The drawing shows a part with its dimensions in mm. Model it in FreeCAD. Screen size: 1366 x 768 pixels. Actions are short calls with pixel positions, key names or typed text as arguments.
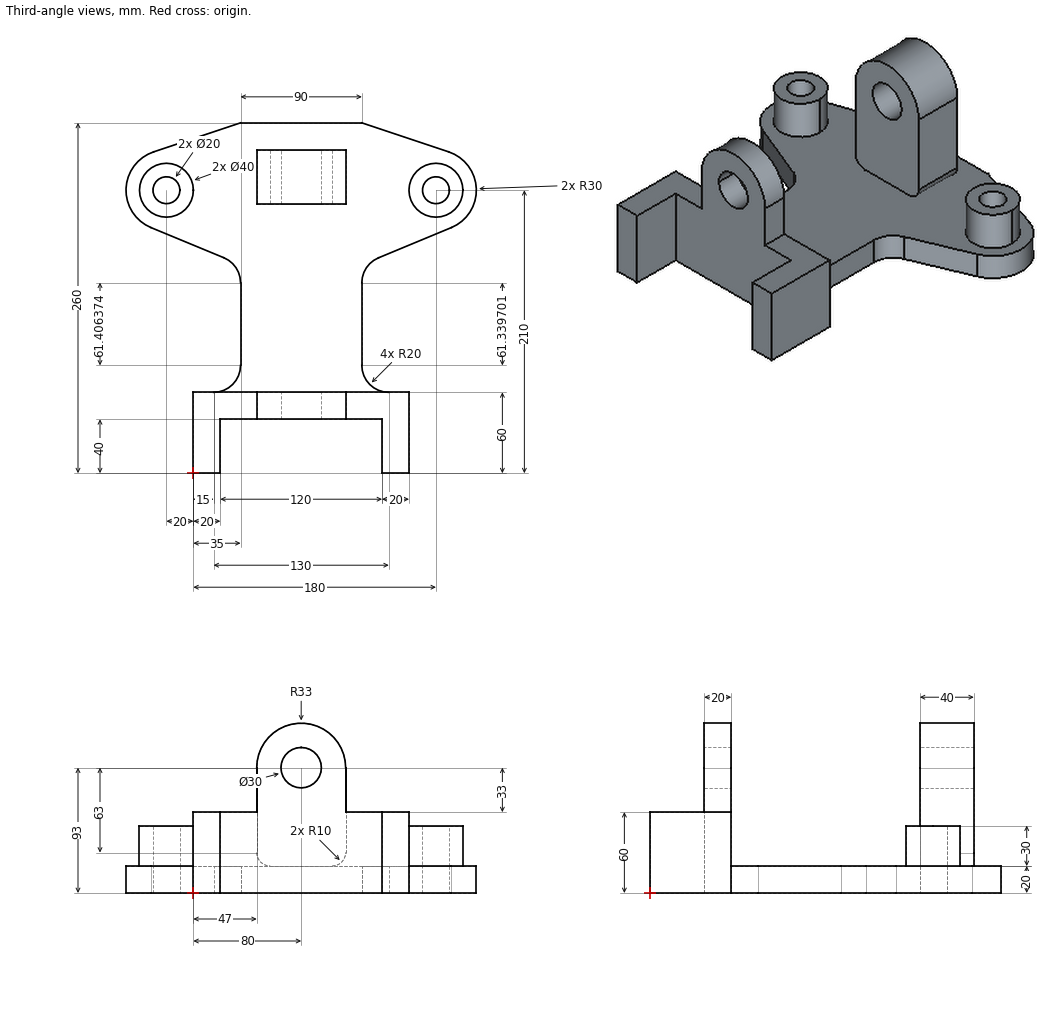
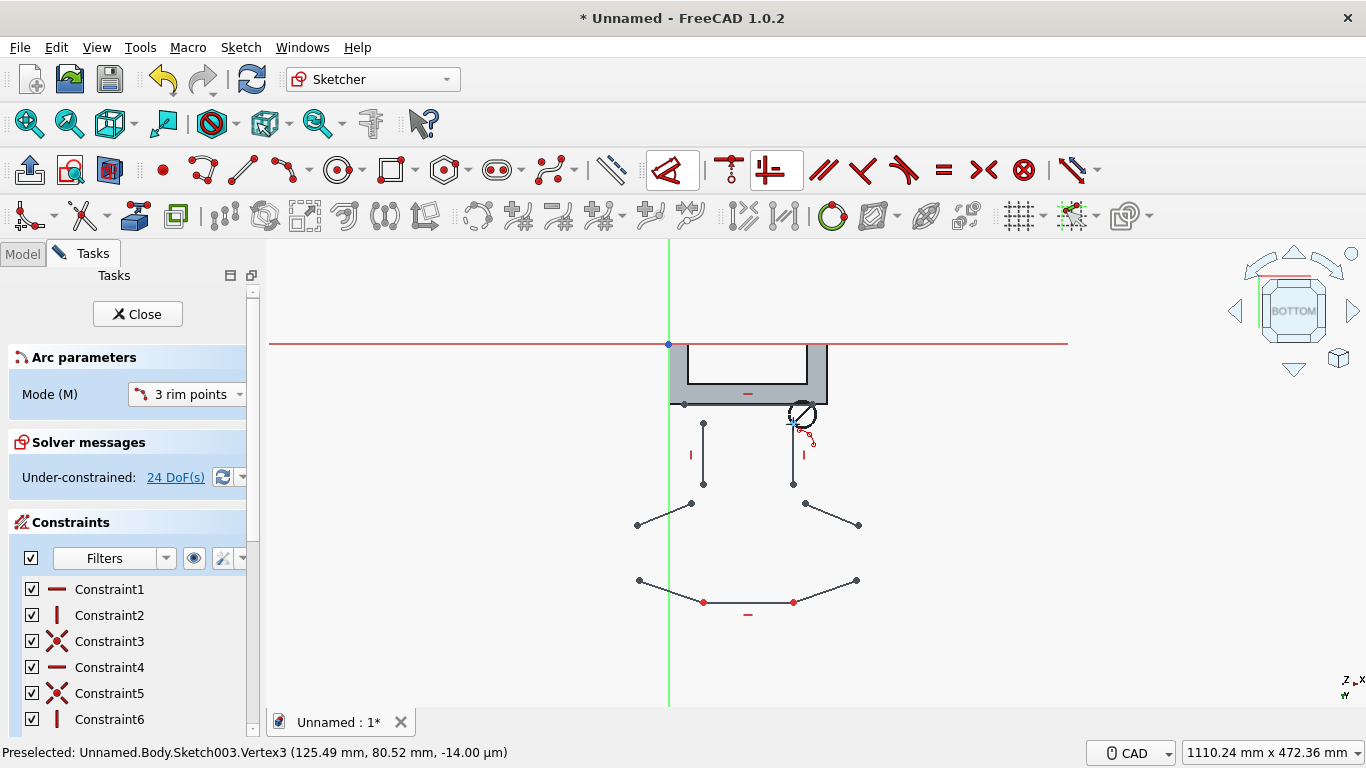
scroll(798, 409, up, 6)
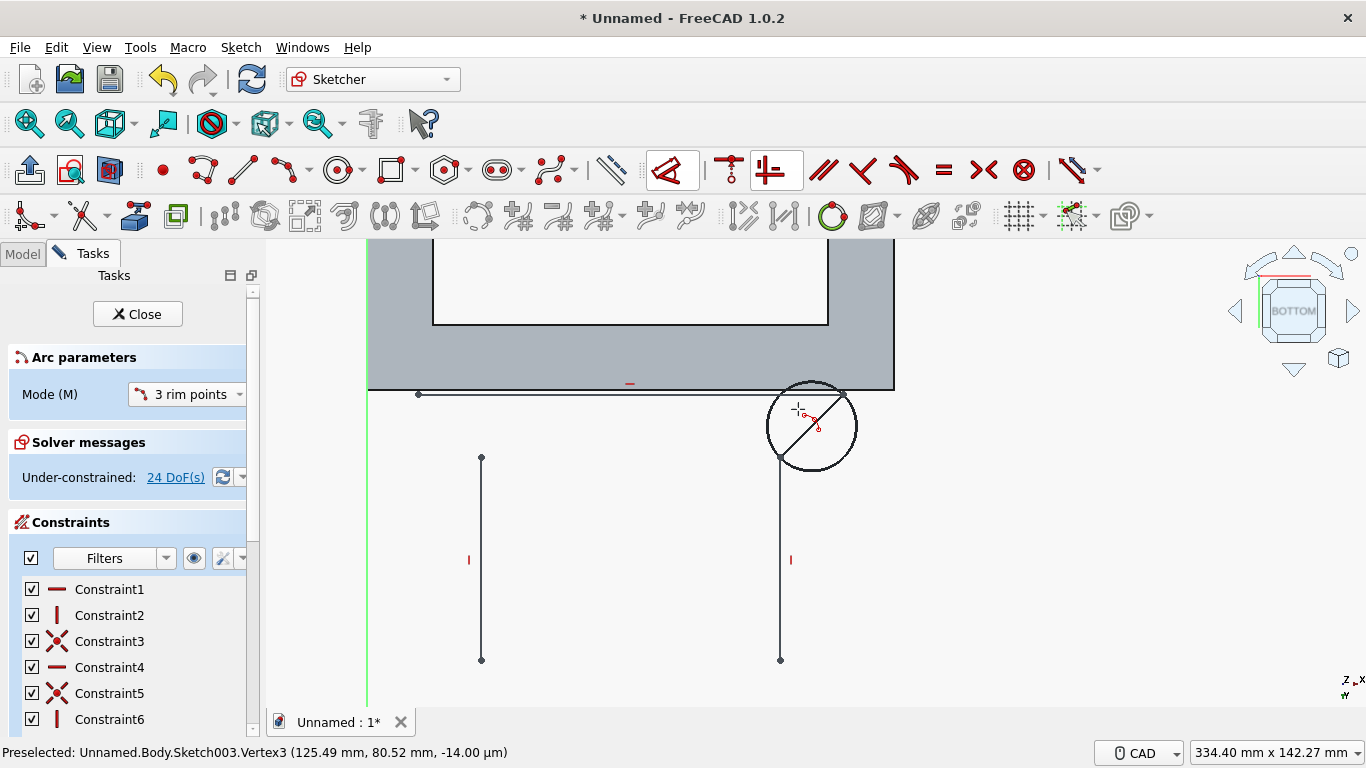
click(798, 410)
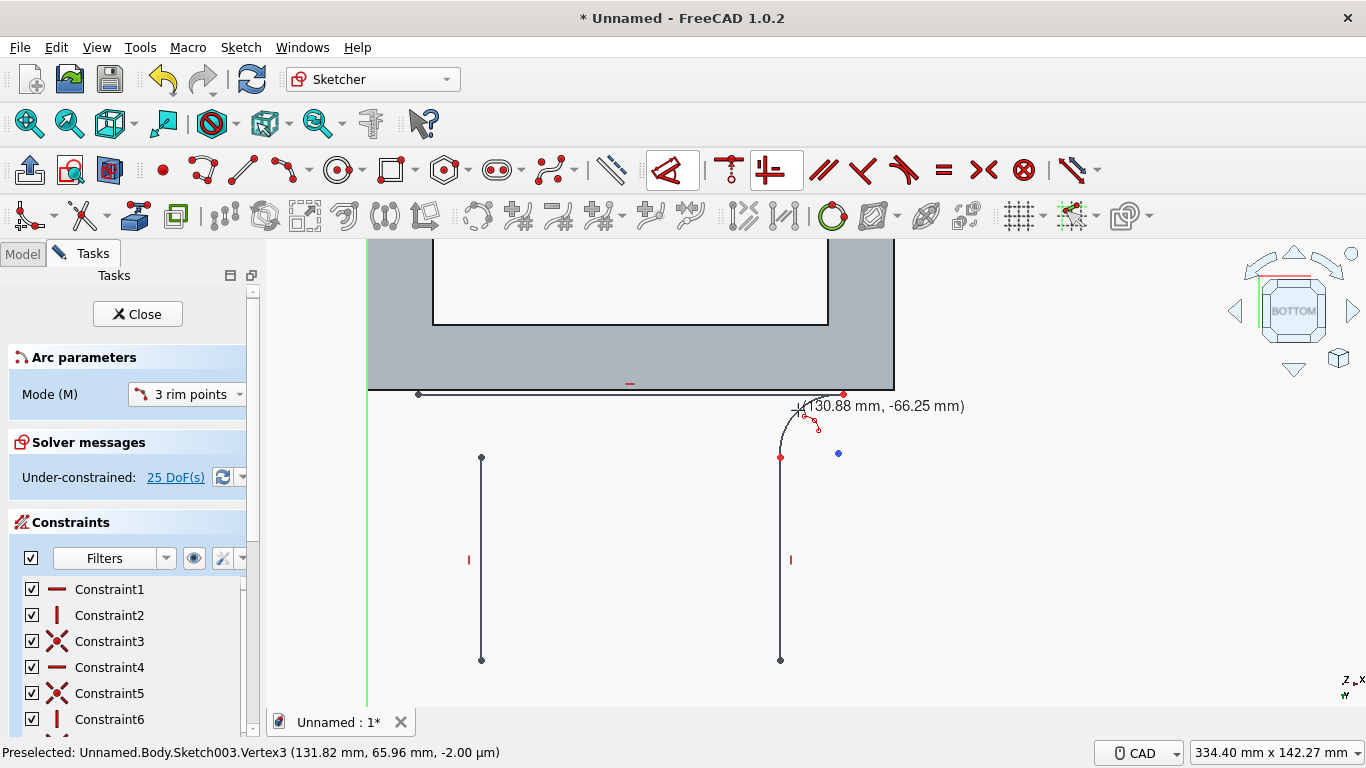
click(780, 660)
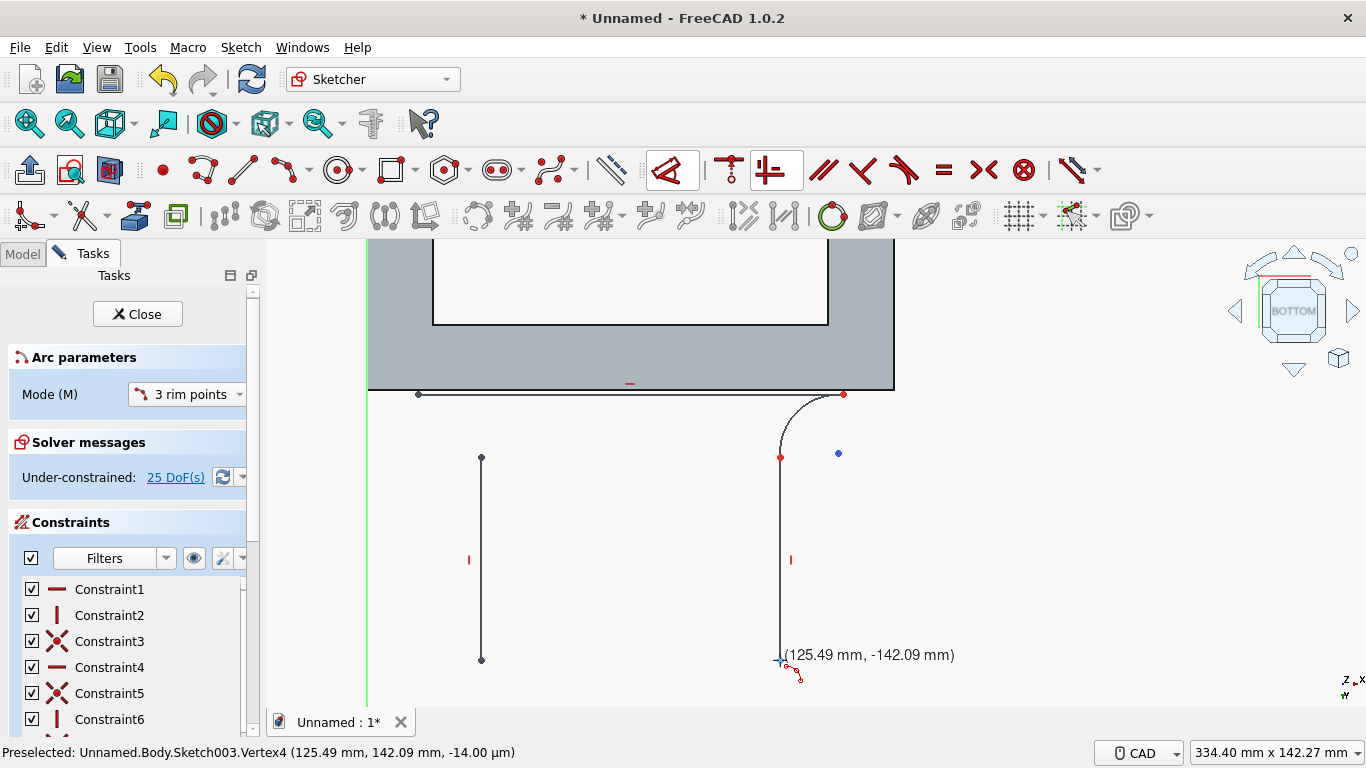
scroll(816, 387, down, 5)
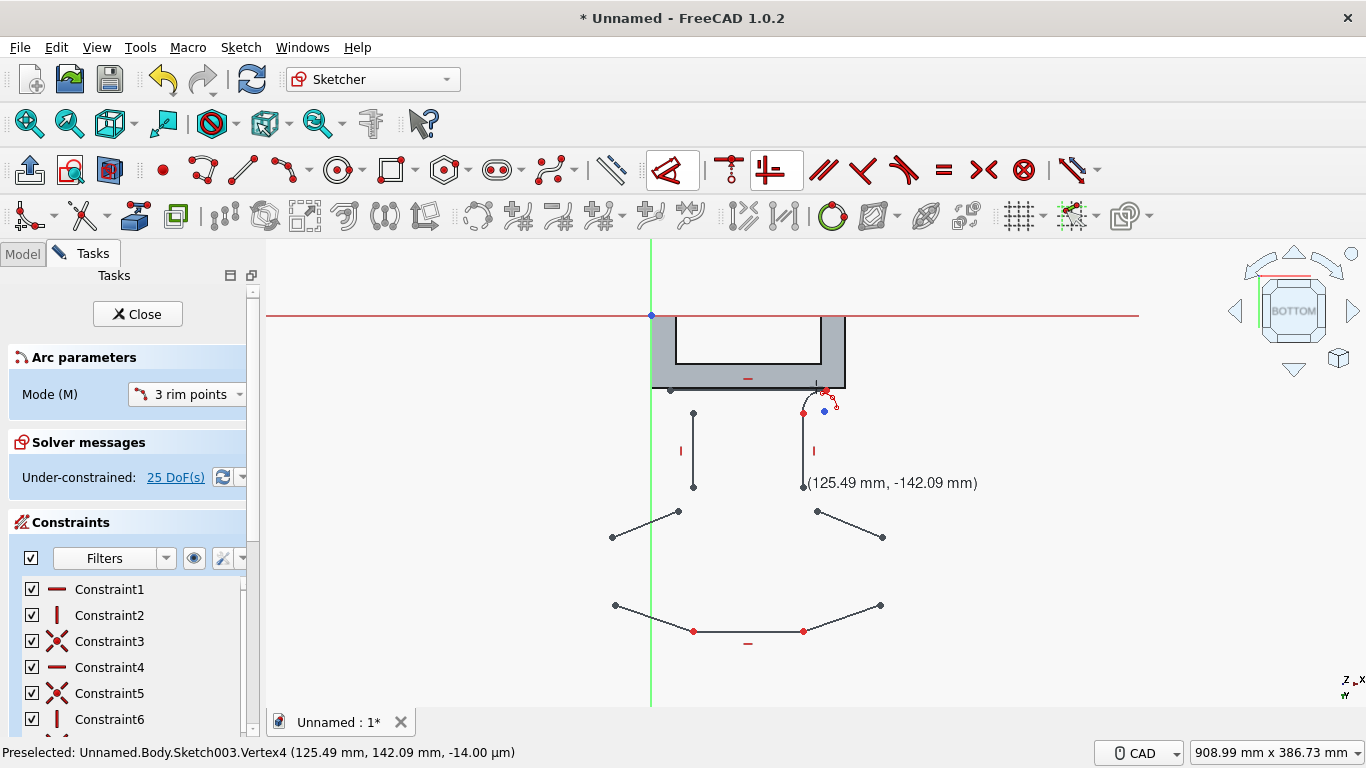
click(818, 511)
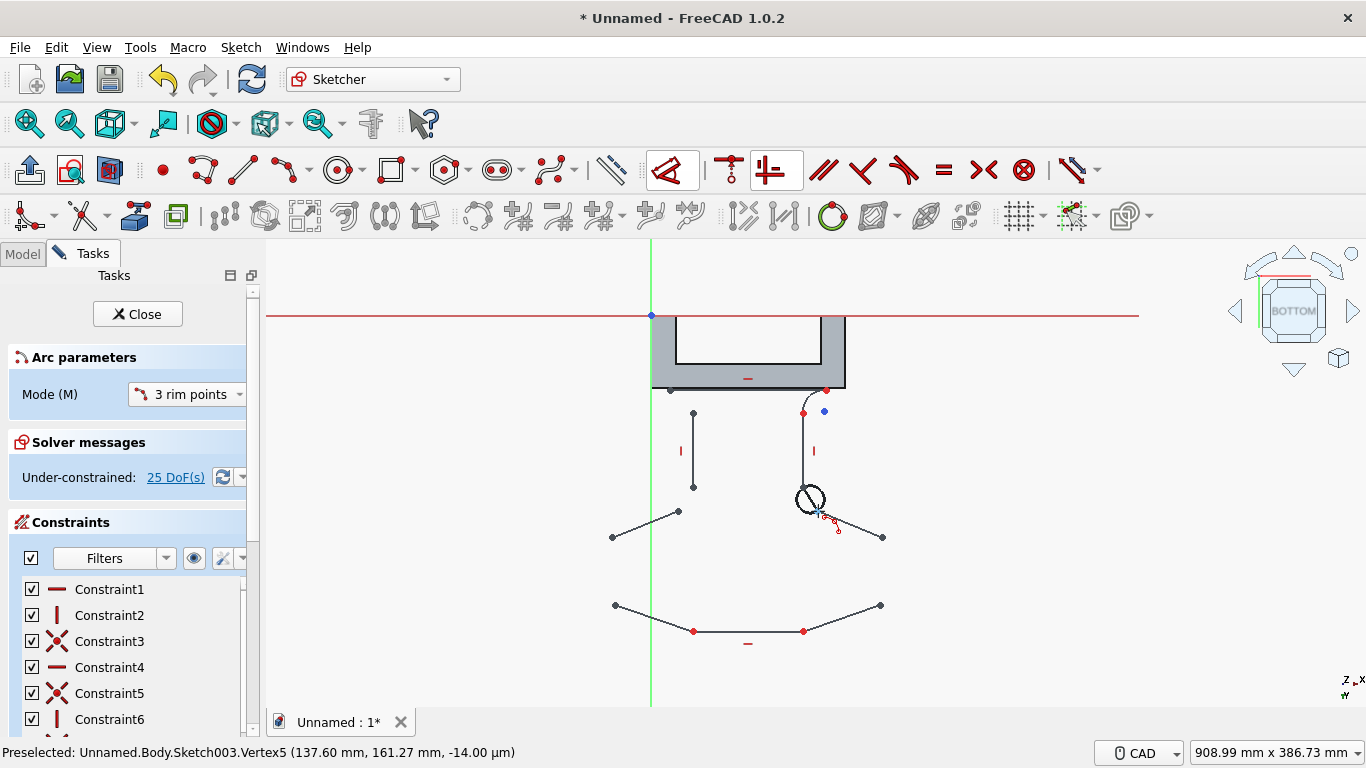
scroll(807, 500, up, 7)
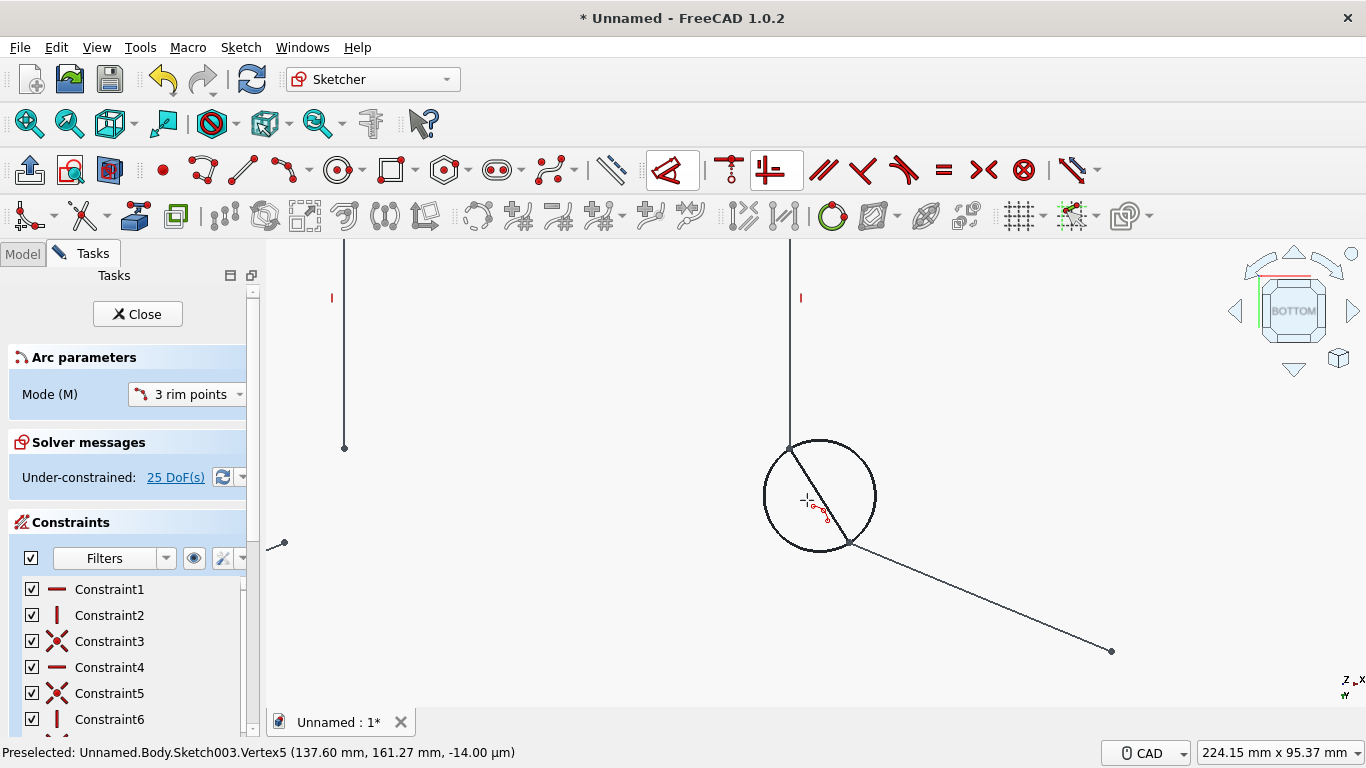
click(804, 500)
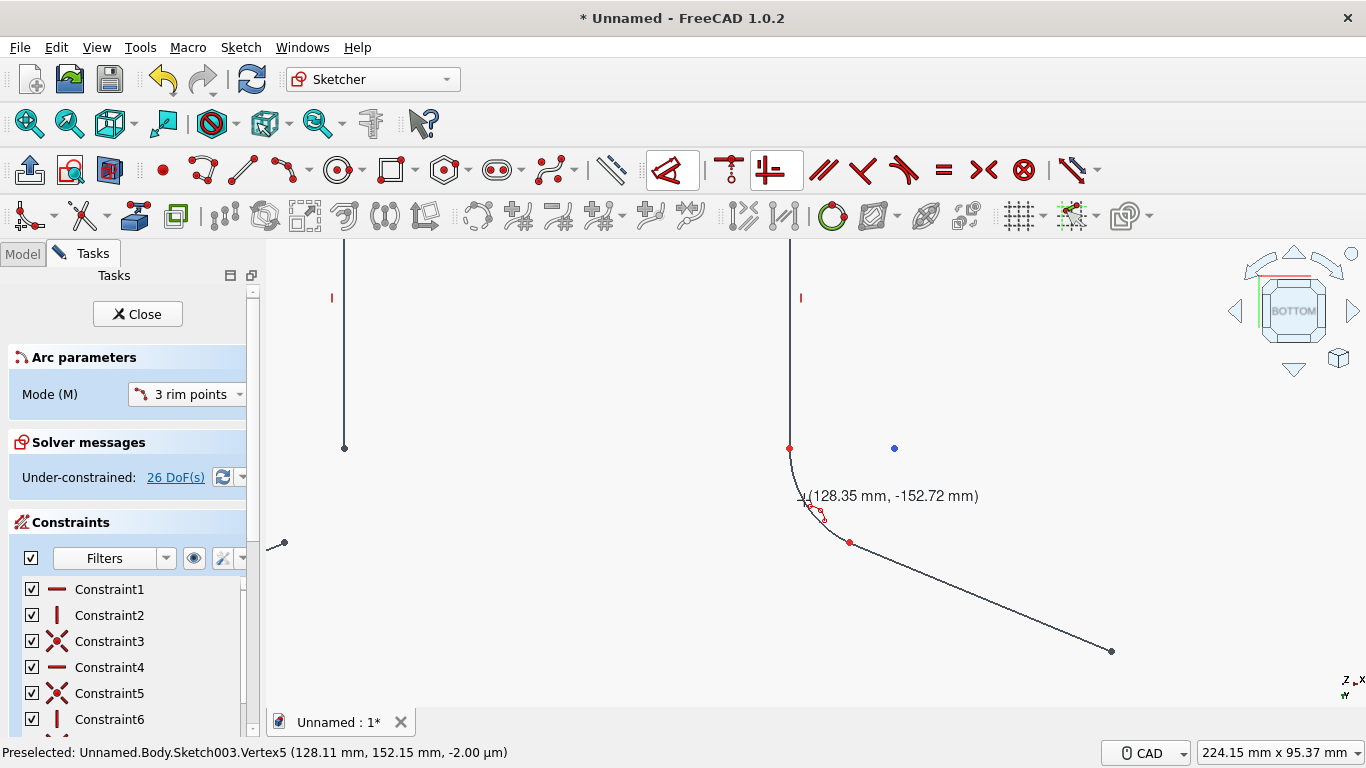
scroll(807, 500, down, 7)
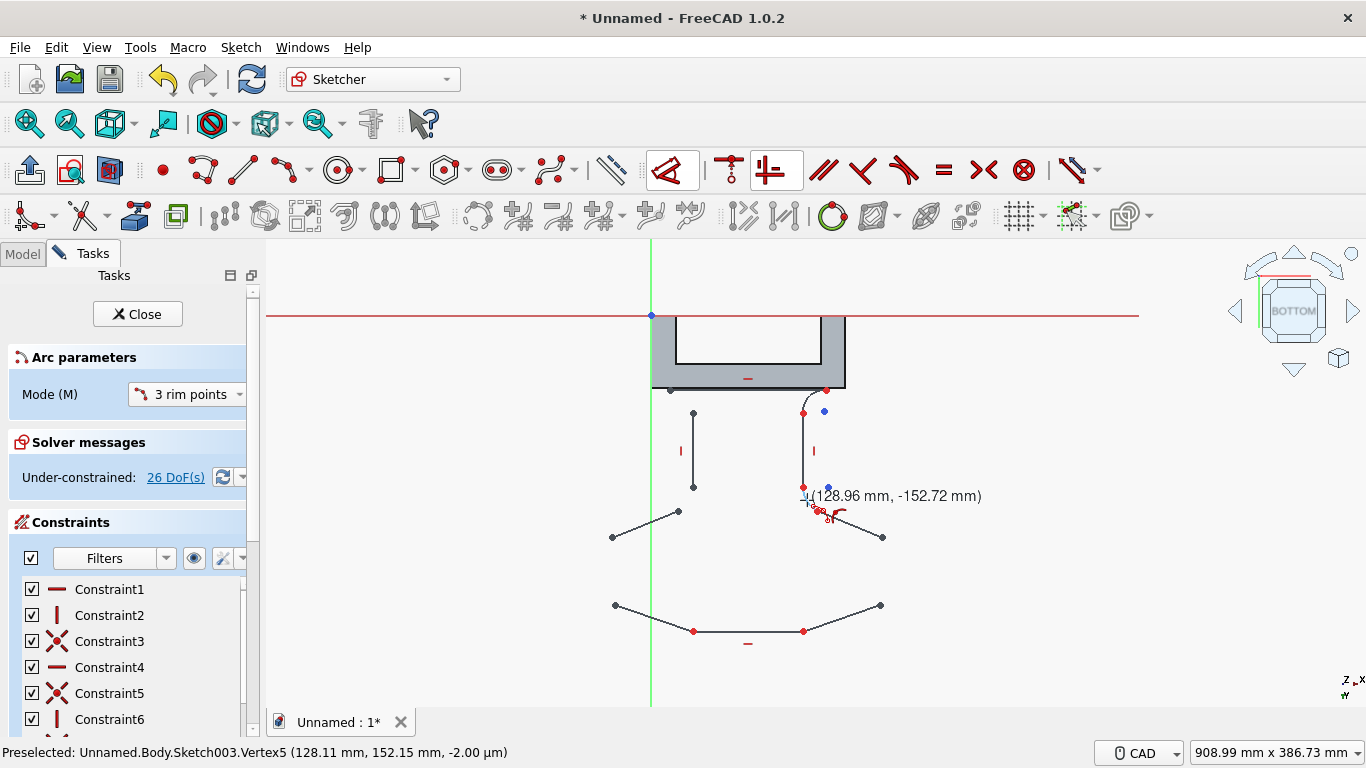
click(883, 538)
click(880, 605)
click(905, 571)